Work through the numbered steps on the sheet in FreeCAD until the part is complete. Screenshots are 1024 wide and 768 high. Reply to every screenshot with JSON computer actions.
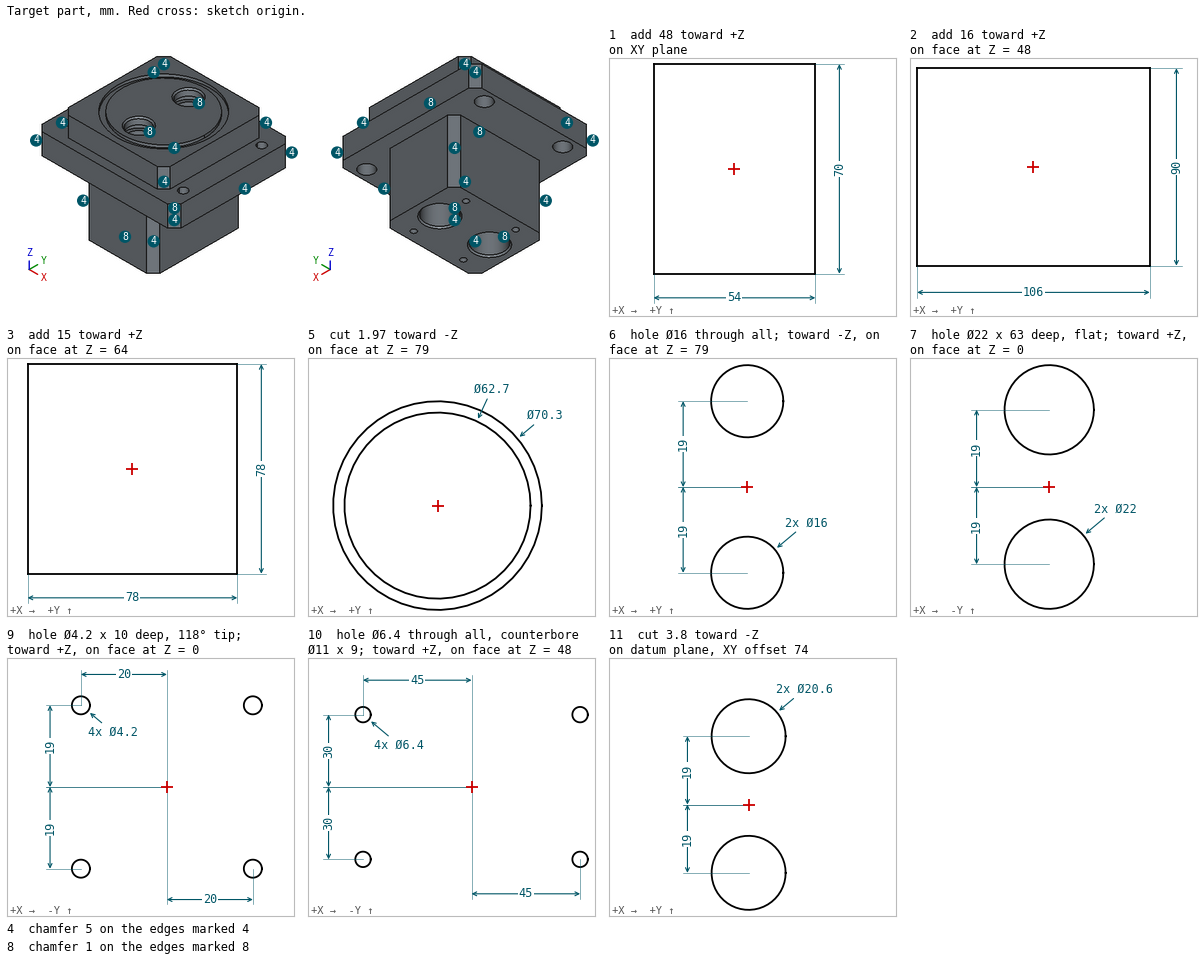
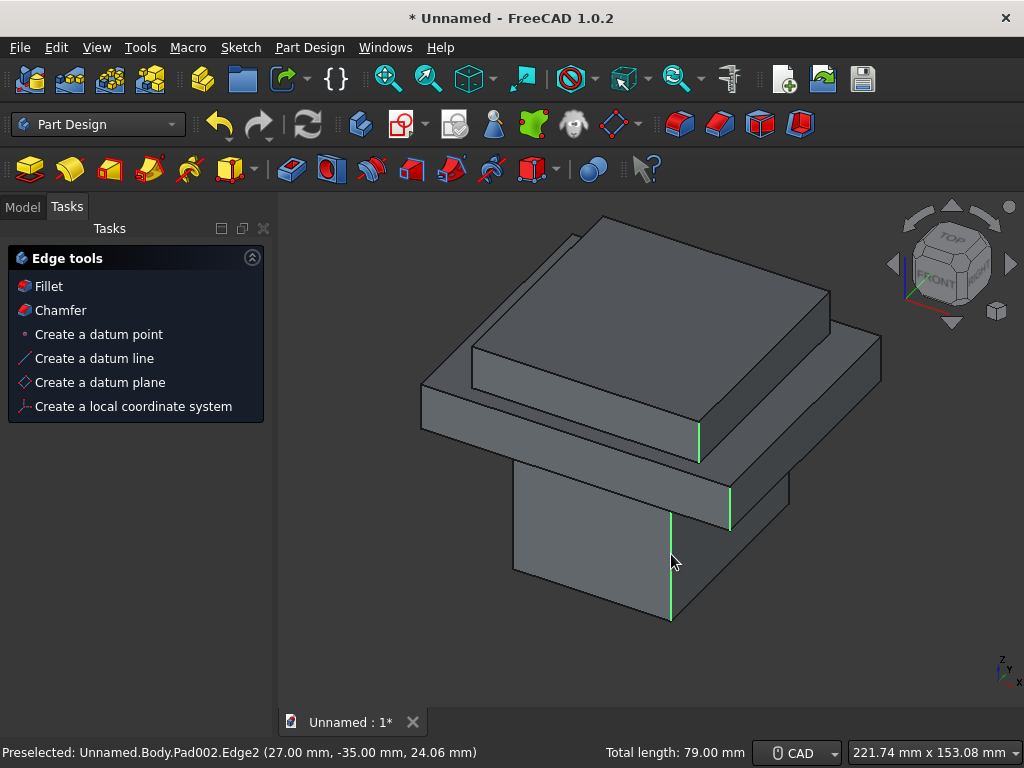
{"action": "key", "text": "0"}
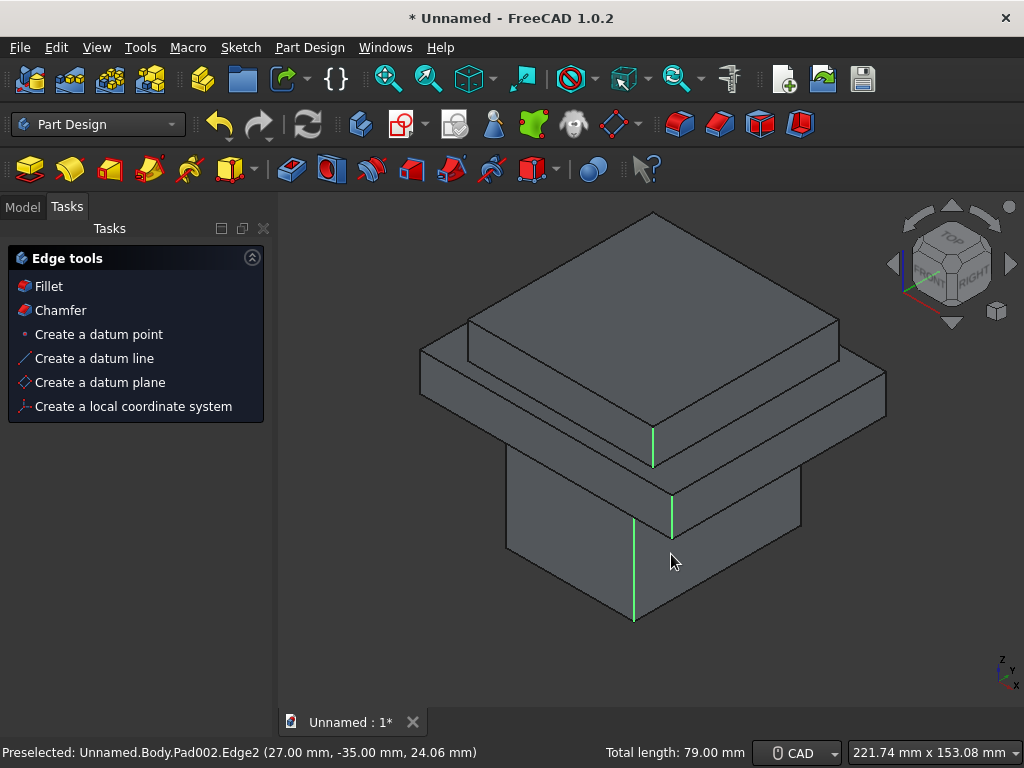
{"action": "left_click", "coordinate": [390, 80]}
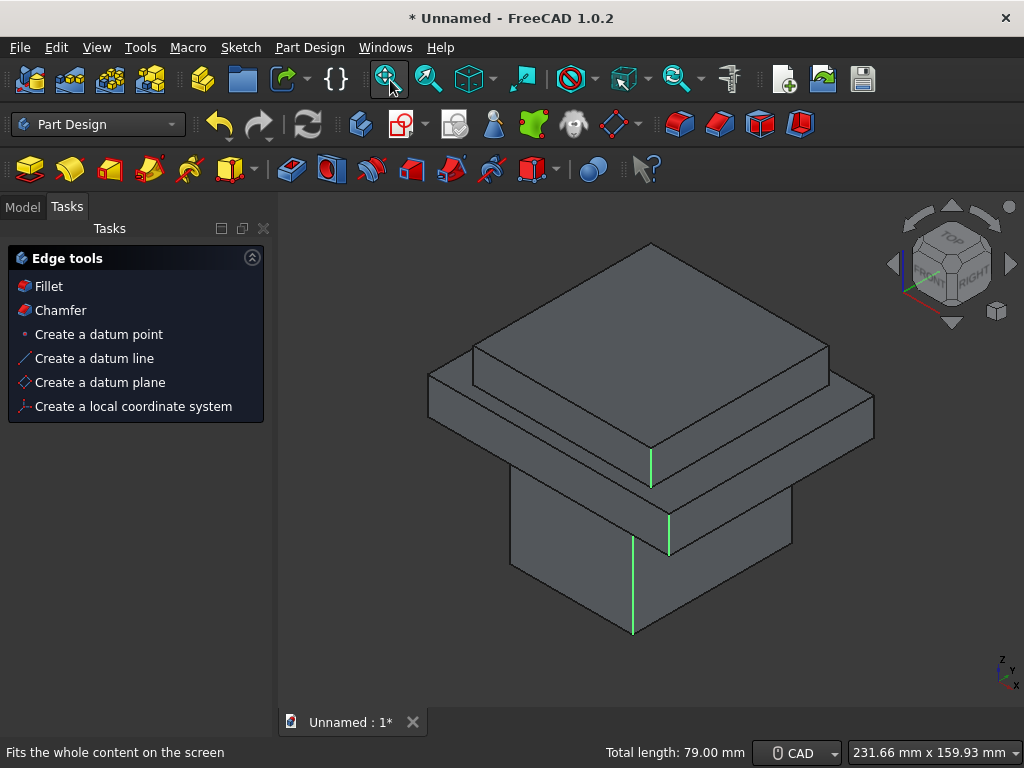
{"action": "key", "text": "2"}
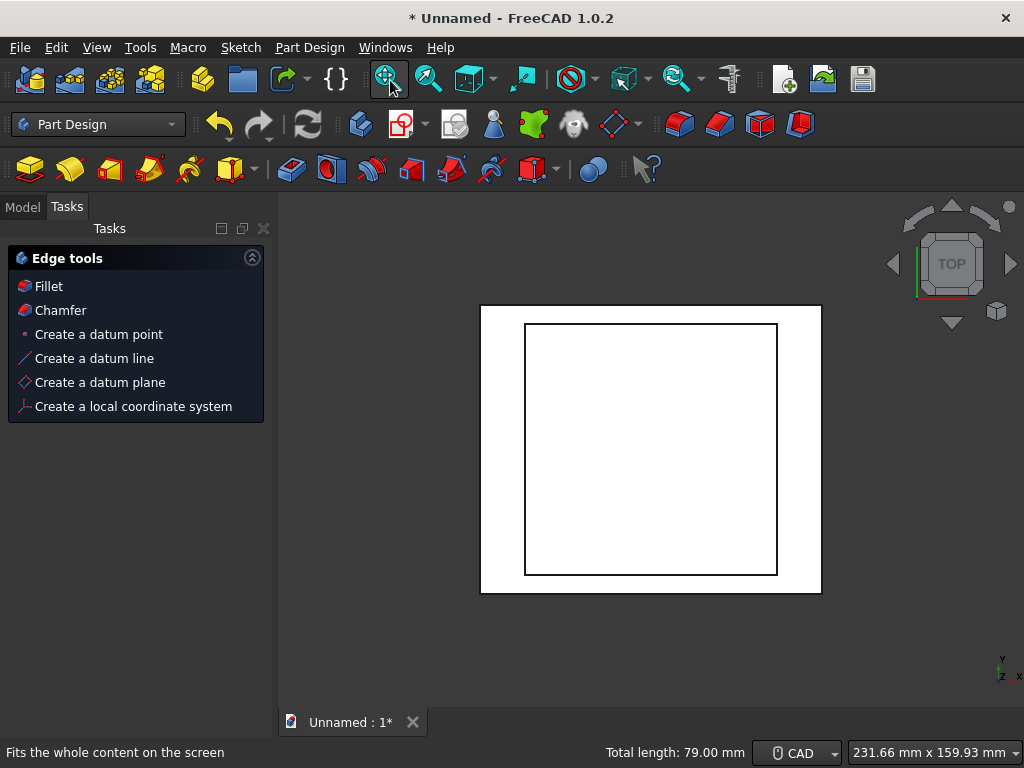
{"action": "key", "text": "1"}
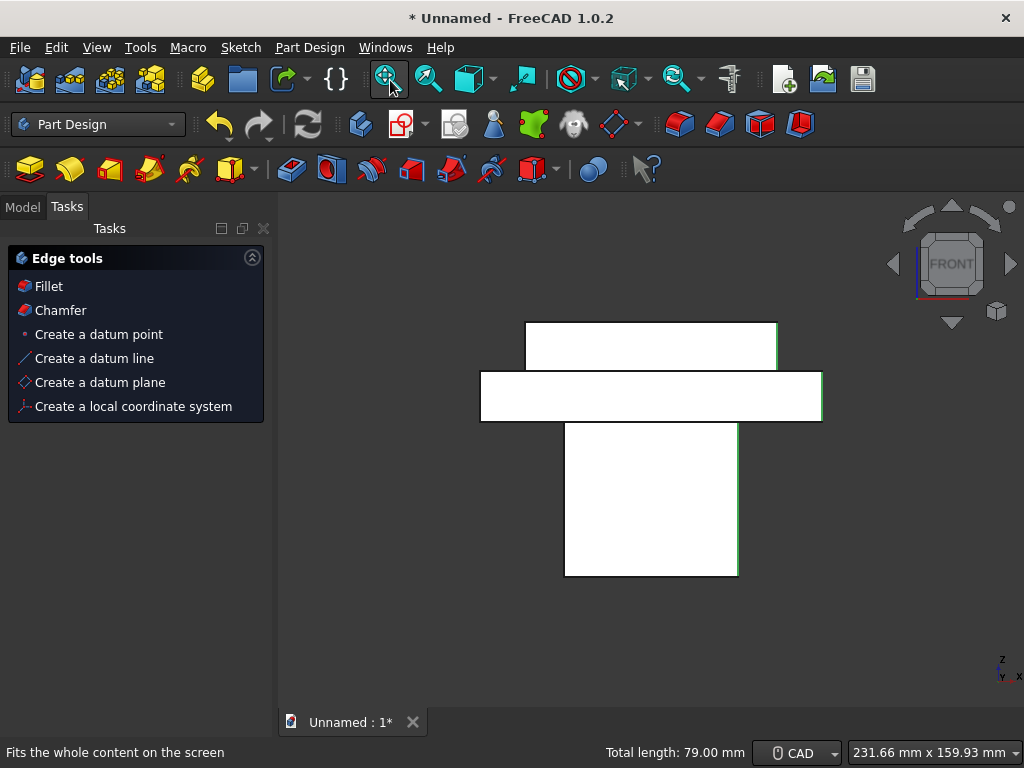
{"action": "left_click", "coordinate": [480, 395], "text": "ctrl"}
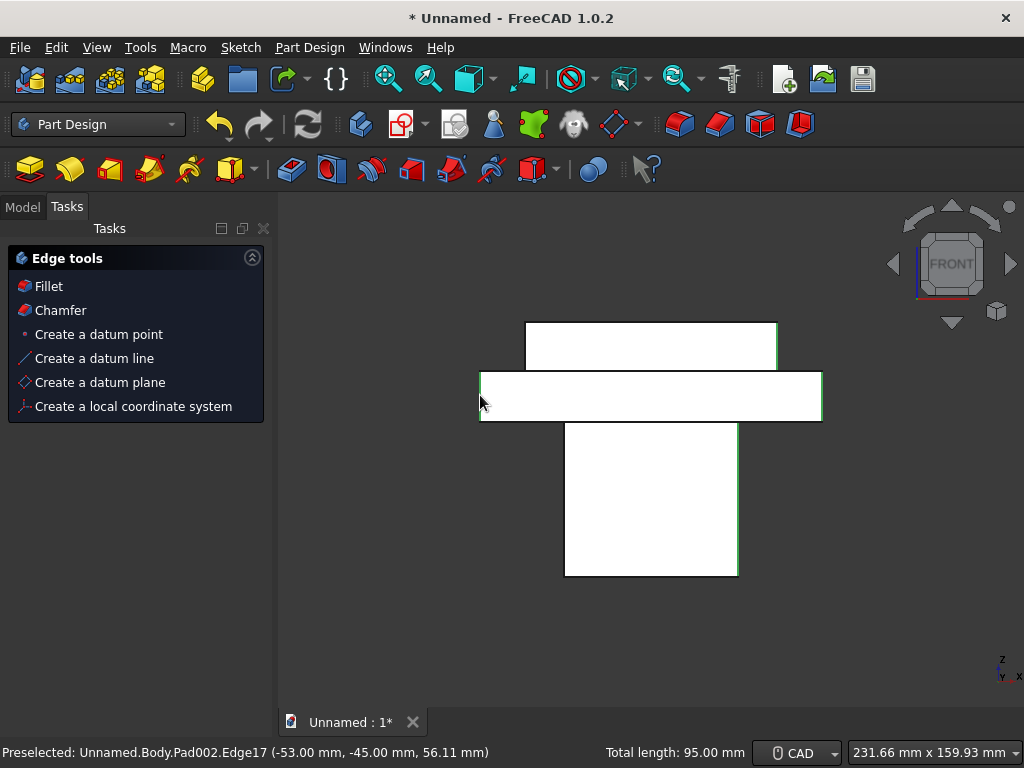
{"action": "left_click", "coordinate": [525, 345], "text": "ctrl"}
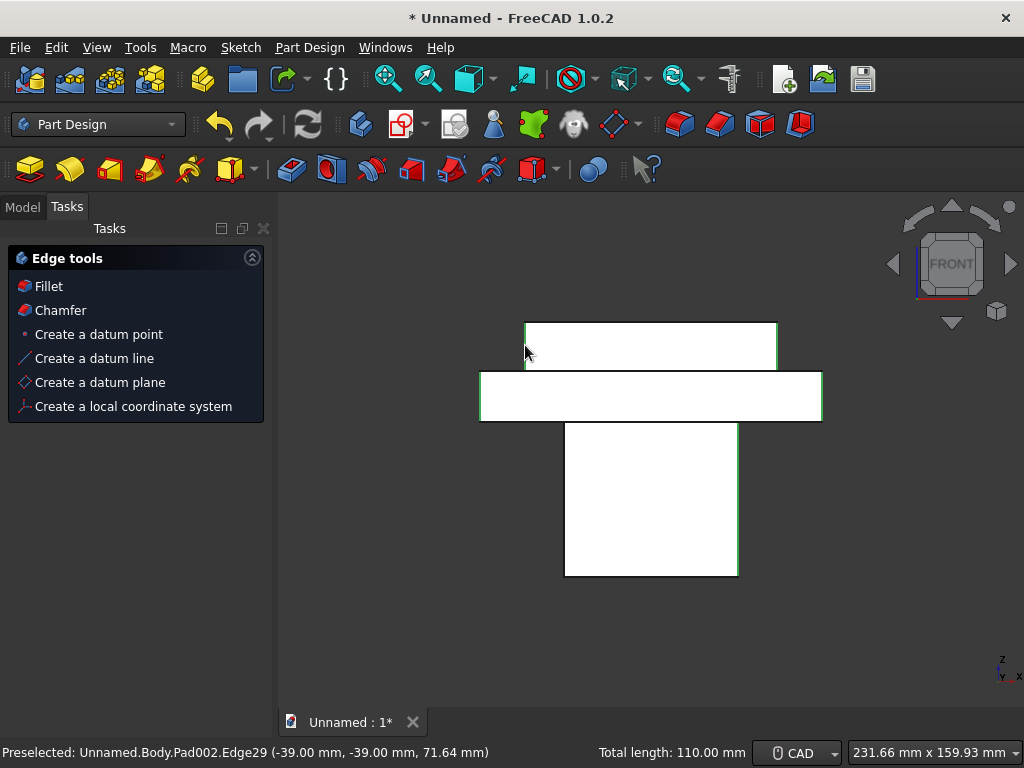
{"action": "left_click", "coordinate": [564, 498], "text": "ctrl"}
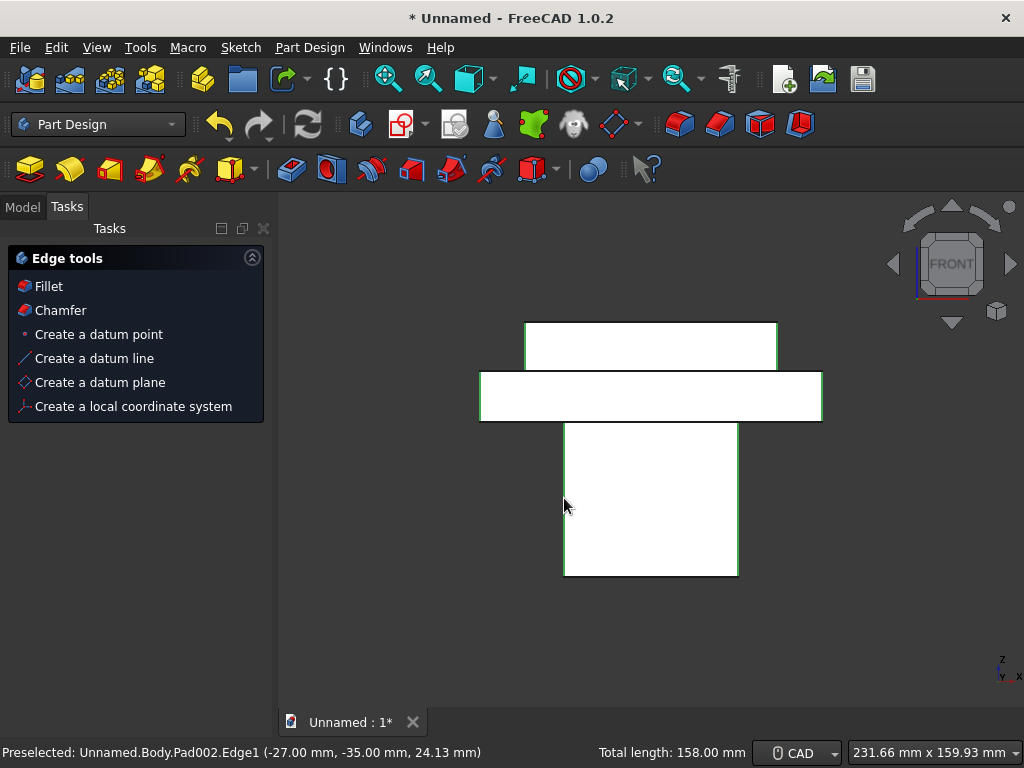
{"action": "key", "text": "3"}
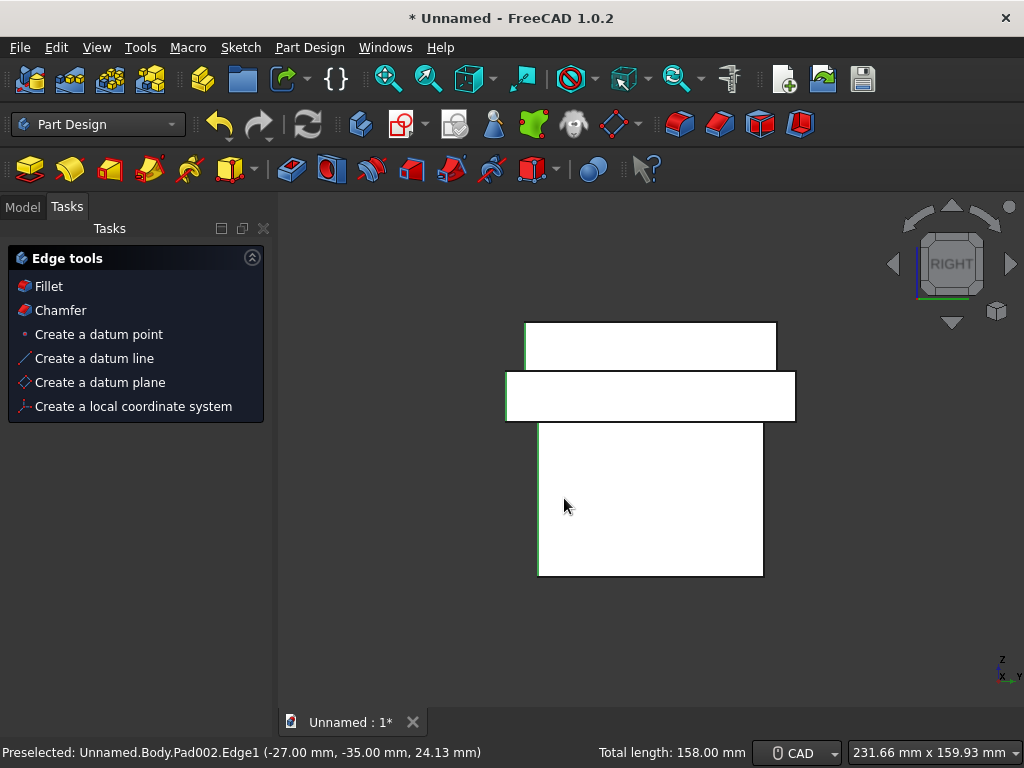
{"action": "left_click", "coordinate": [796, 395], "text": "ctrl"}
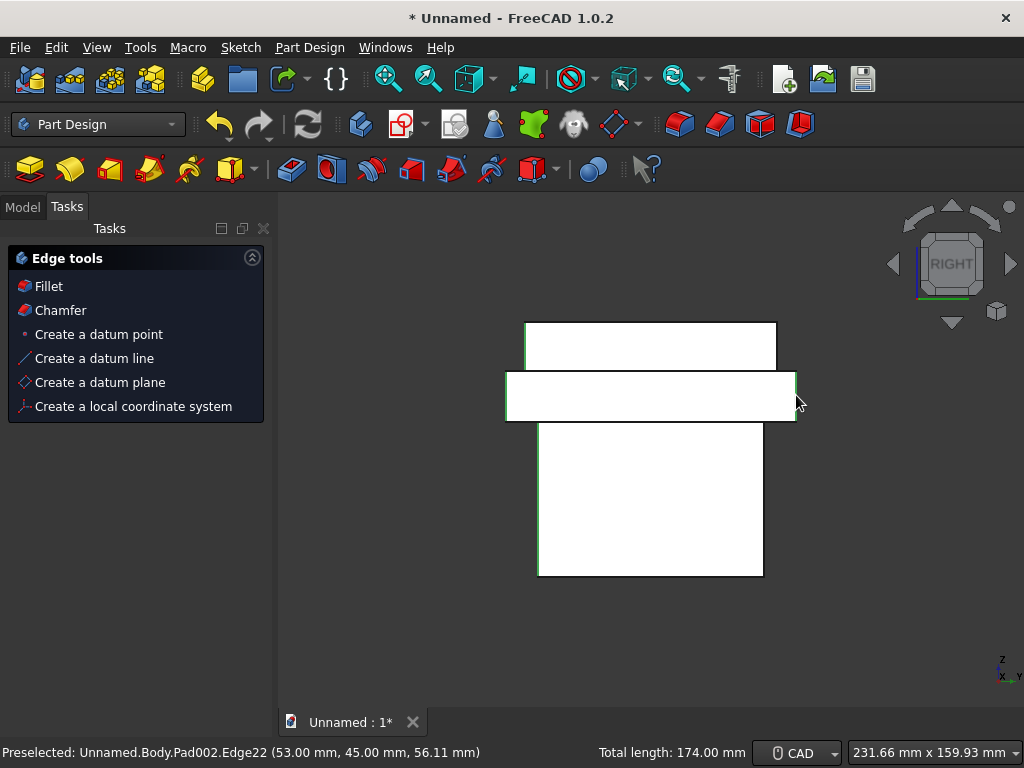
{"action": "left_click", "coordinate": [777, 345], "text": "ctrl"}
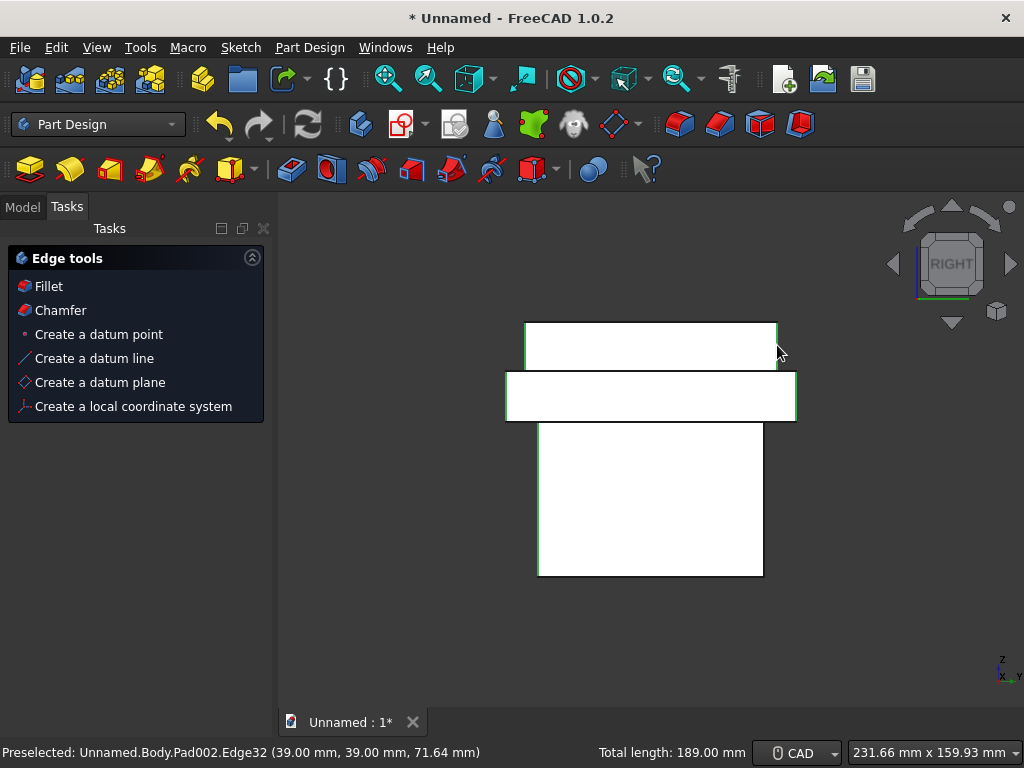
{"action": "left_click", "coordinate": [764, 498], "text": "ctrl"}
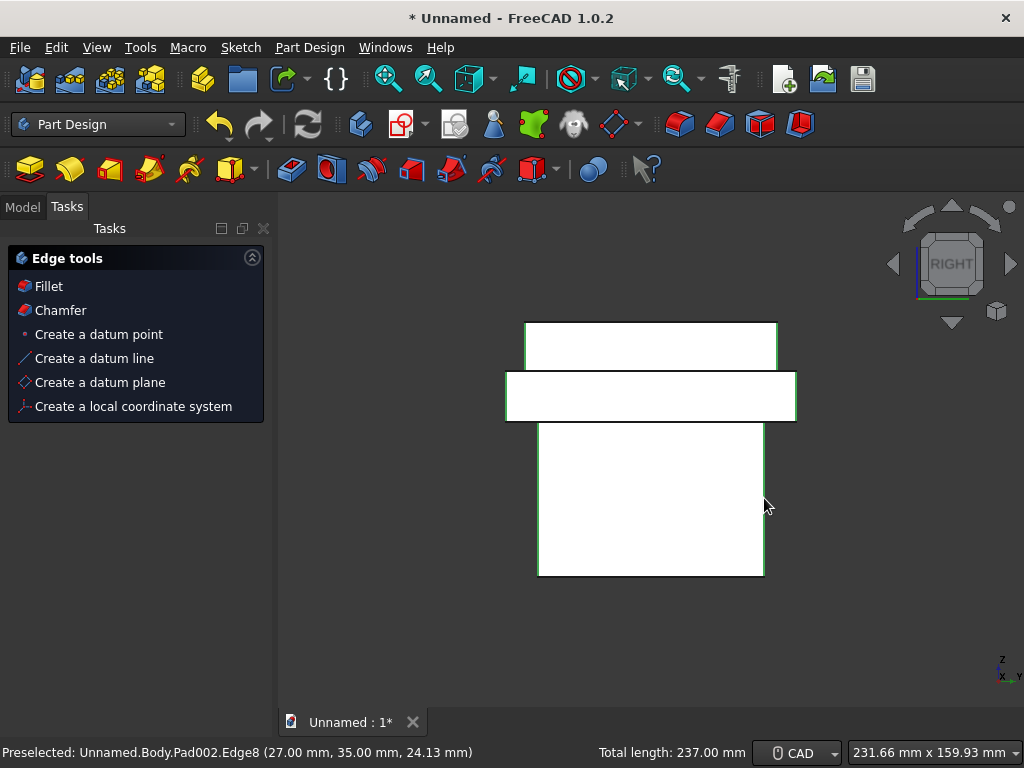
{"action": "key", "text": "5"}